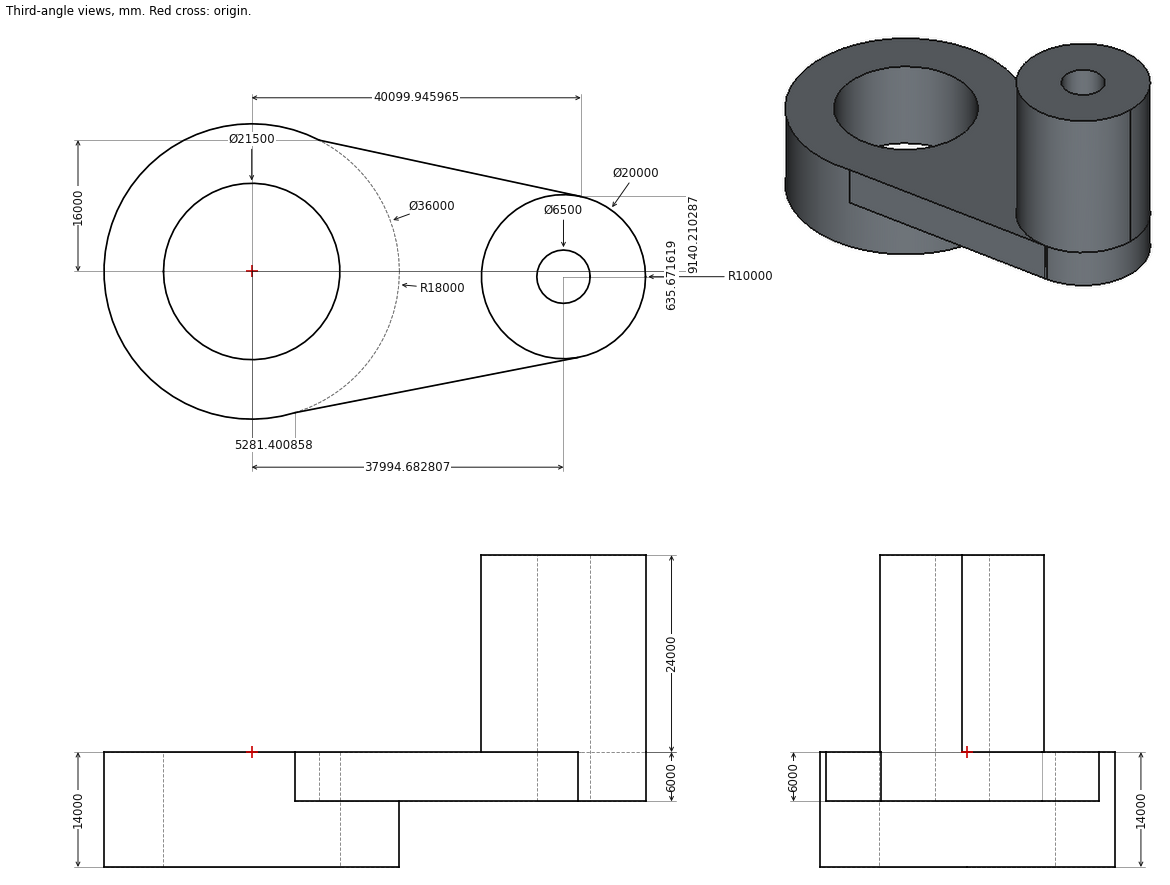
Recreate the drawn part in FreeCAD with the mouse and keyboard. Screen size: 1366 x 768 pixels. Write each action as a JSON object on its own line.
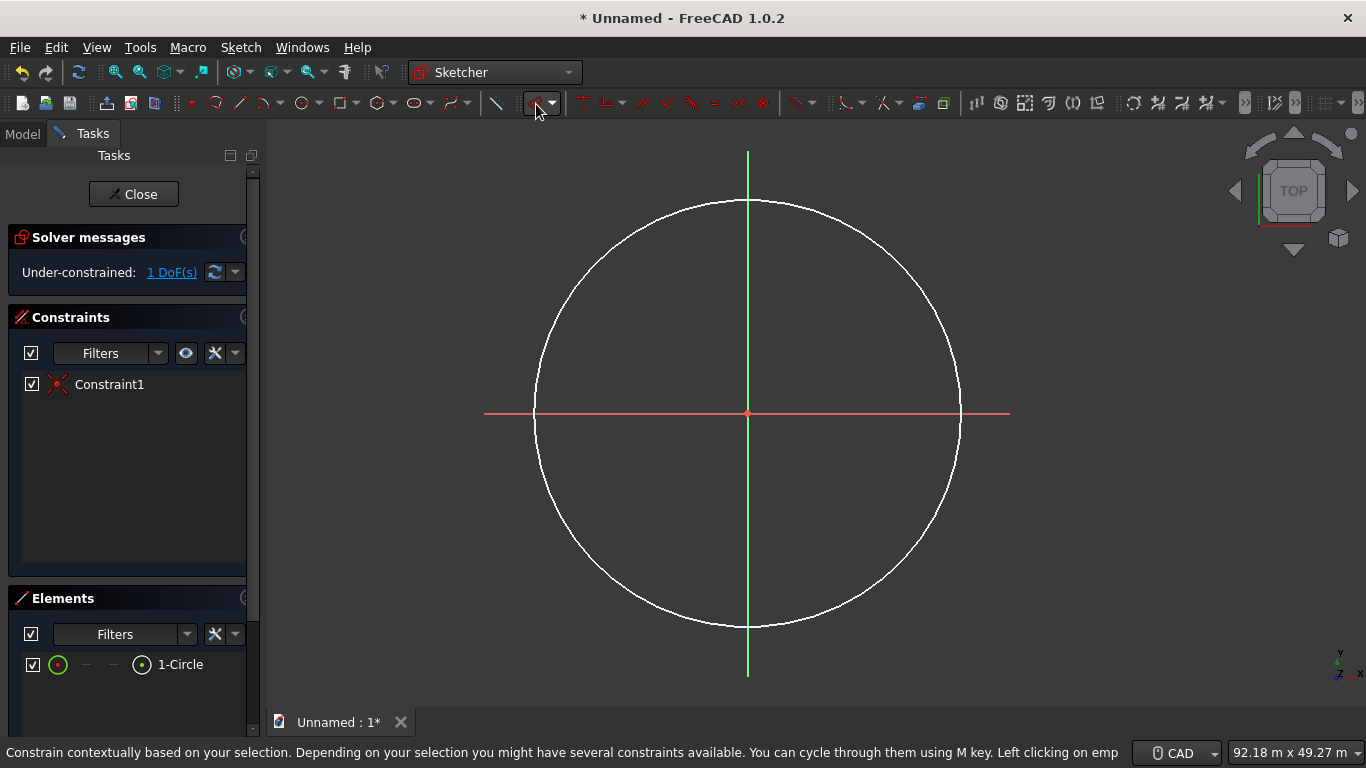
{"action": "left_click", "coordinate": [898, 262]}
{"action": "left_click", "coordinate": [921, 239]}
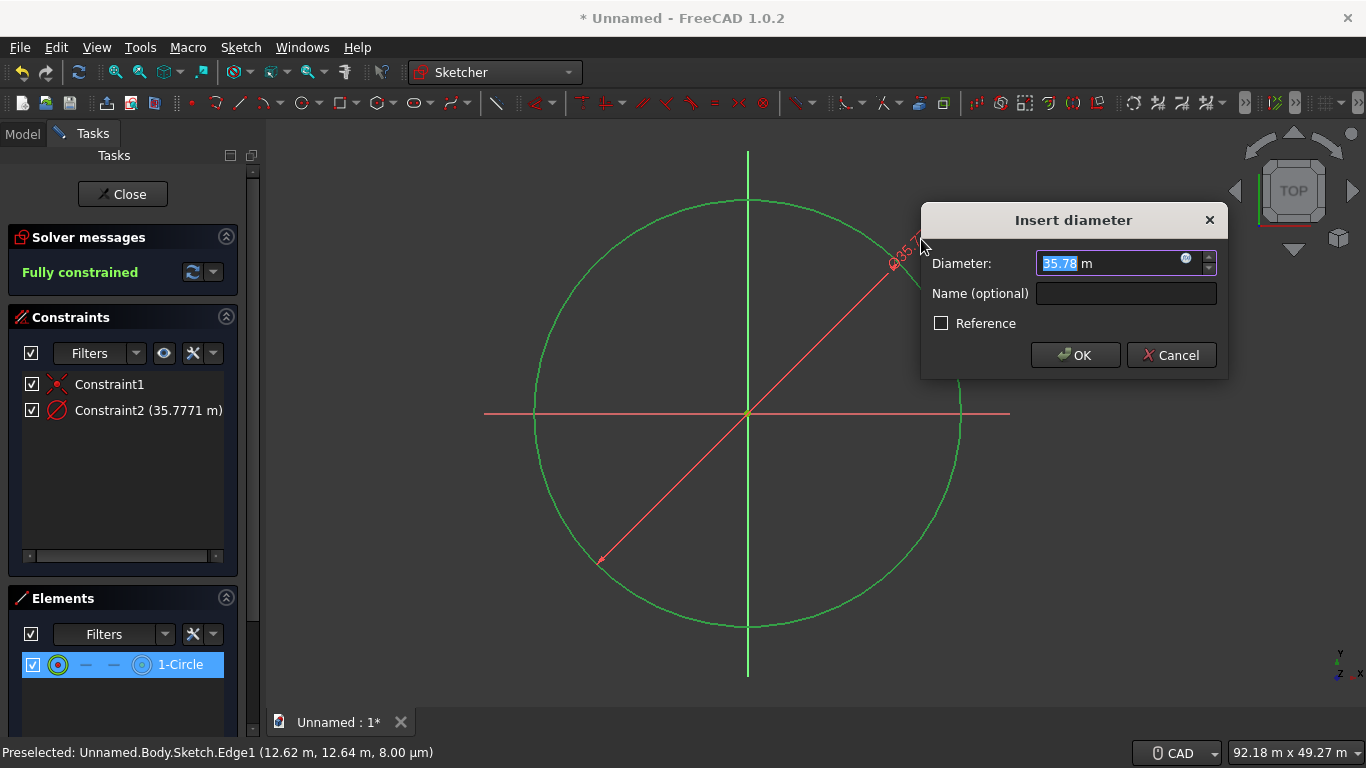
{"action": "key", "text": "ctrl+a"}
{"action": "type", "text": "36000 mm"}
{"action": "key", "text": "Return"}
{"action": "key", "text": "Escape"}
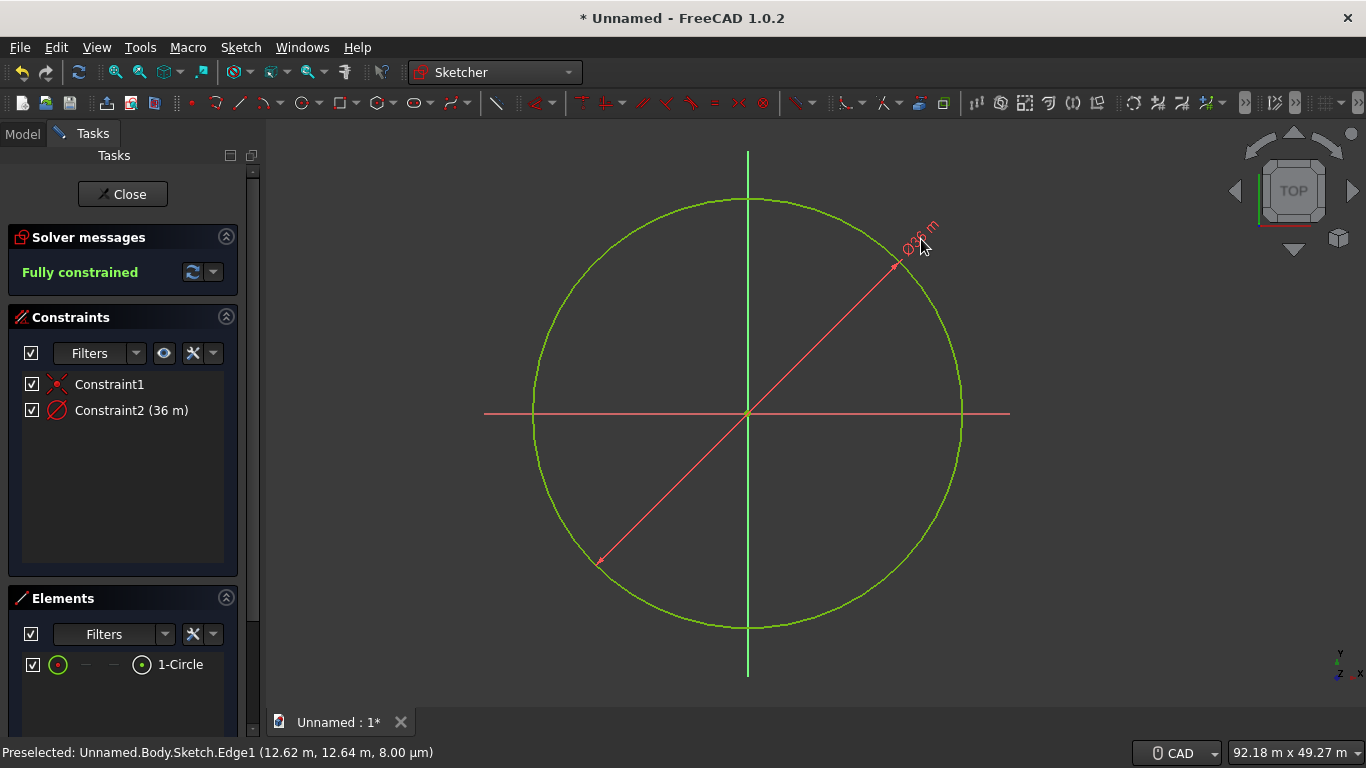
{"action": "left_click", "coordinate": [123, 194]}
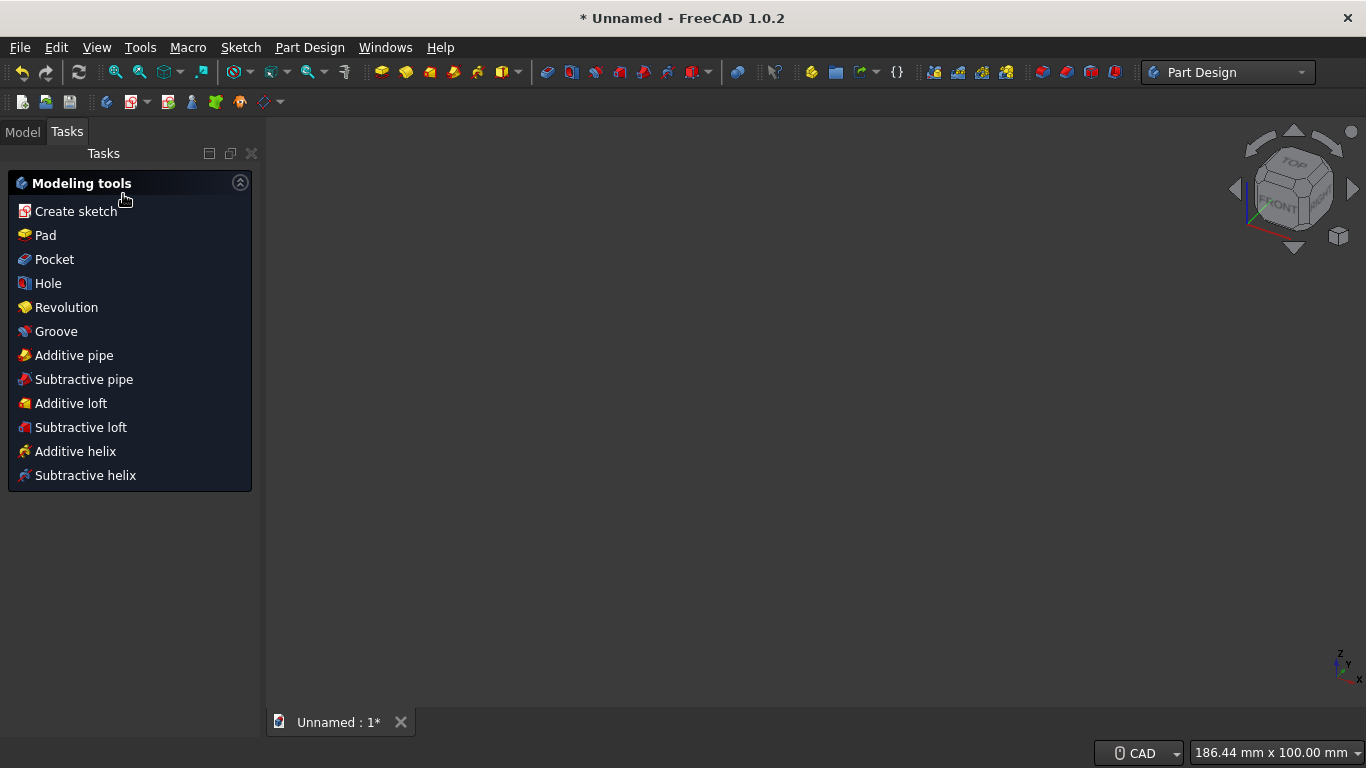
{"action": "left_click", "coordinate": [382, 72]}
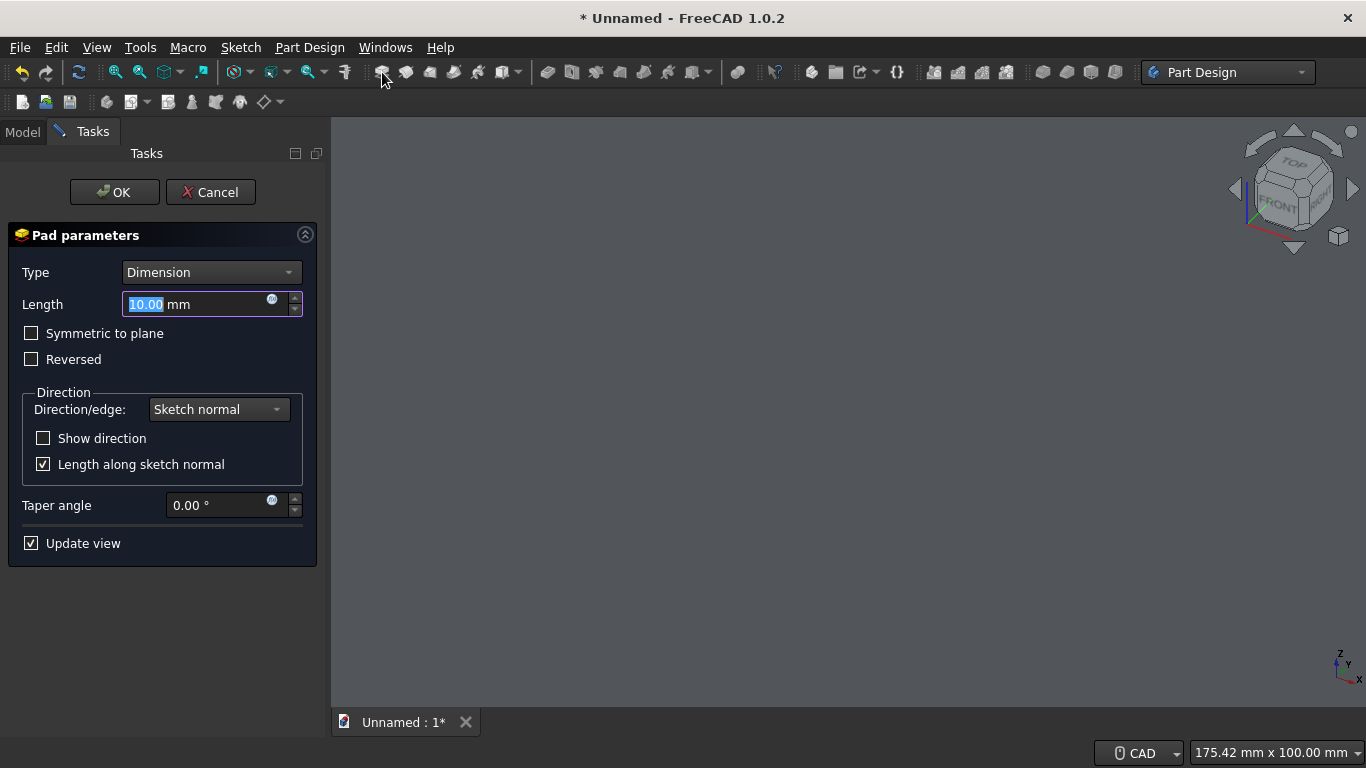
{"action": "type", "text": "14000"}
{"action": "key", "text": "Tab"}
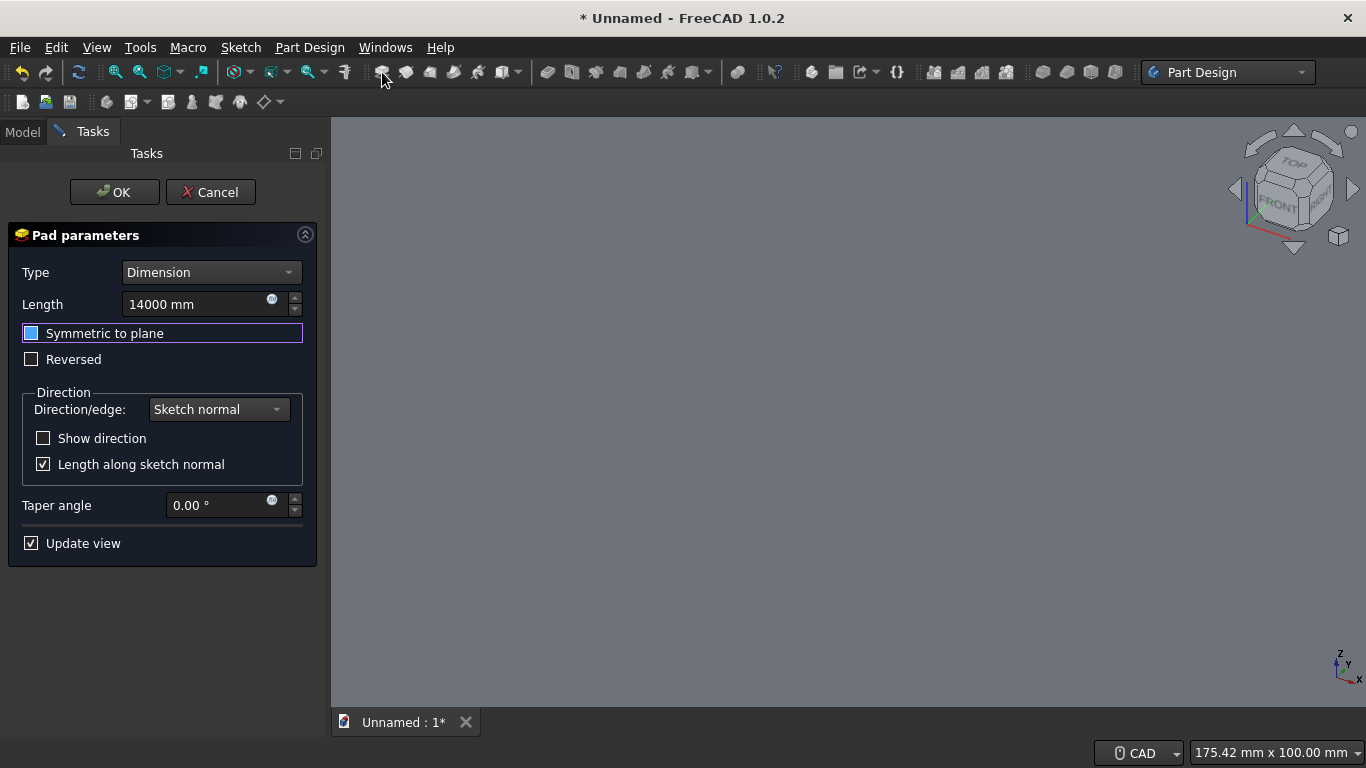
{"action": "left_click", "coordinate": [30, 359]}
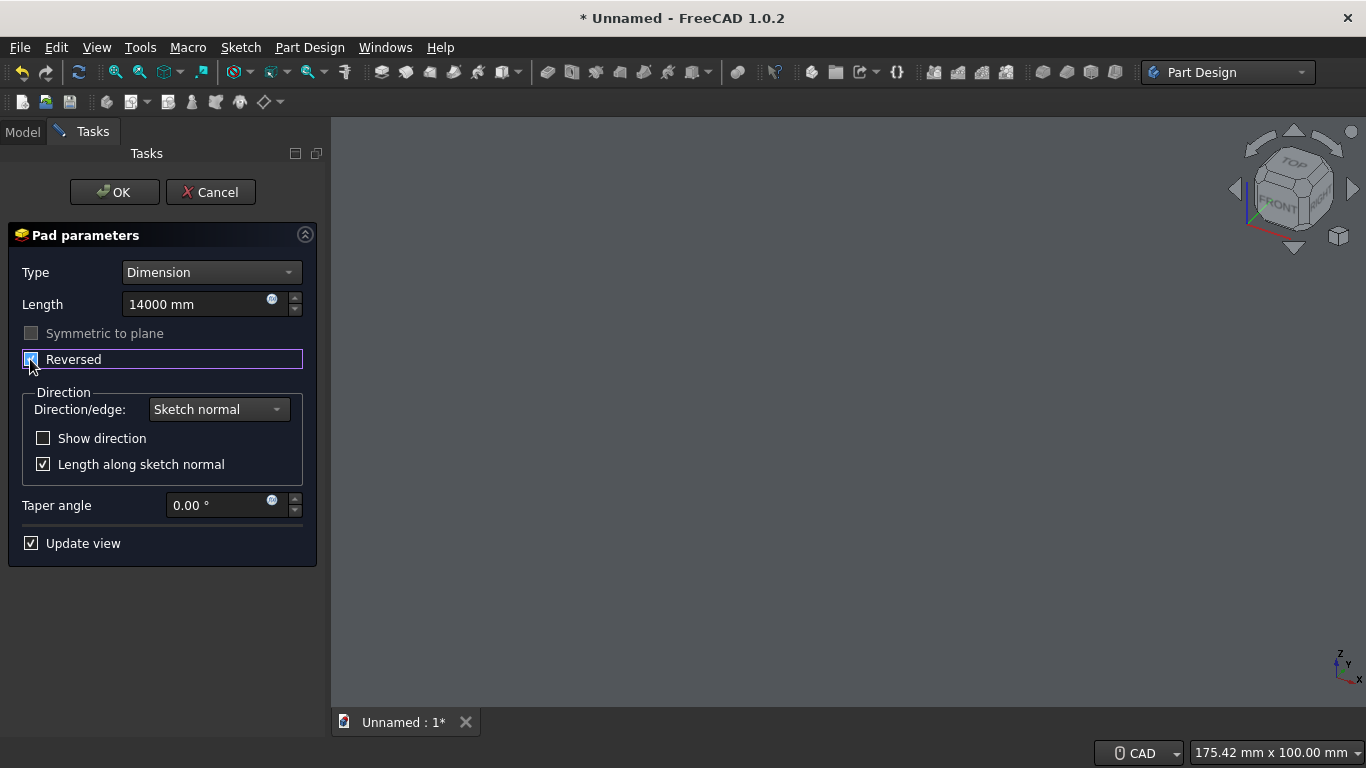
{"action": "left_click", "coordinate": [115, 192]}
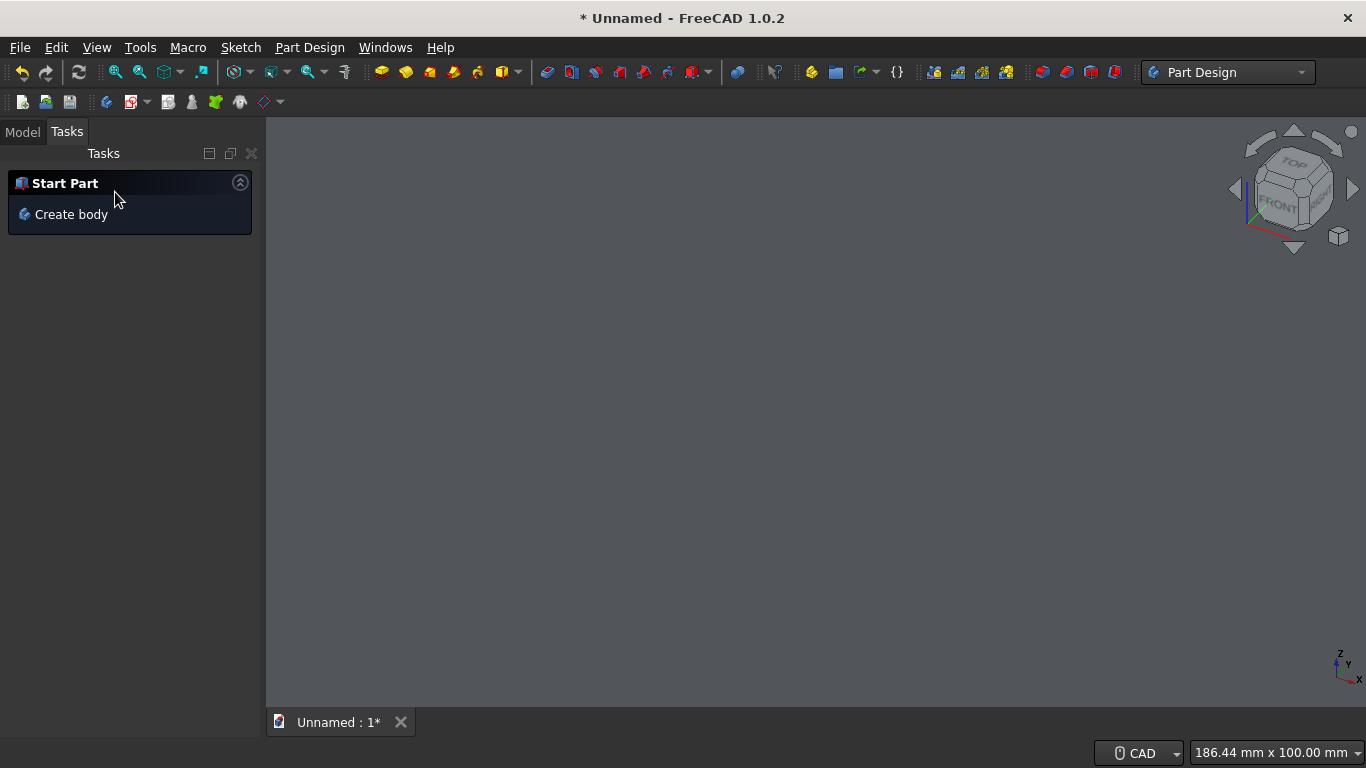
{"action": "left_click", "coordinate": [116, 72]}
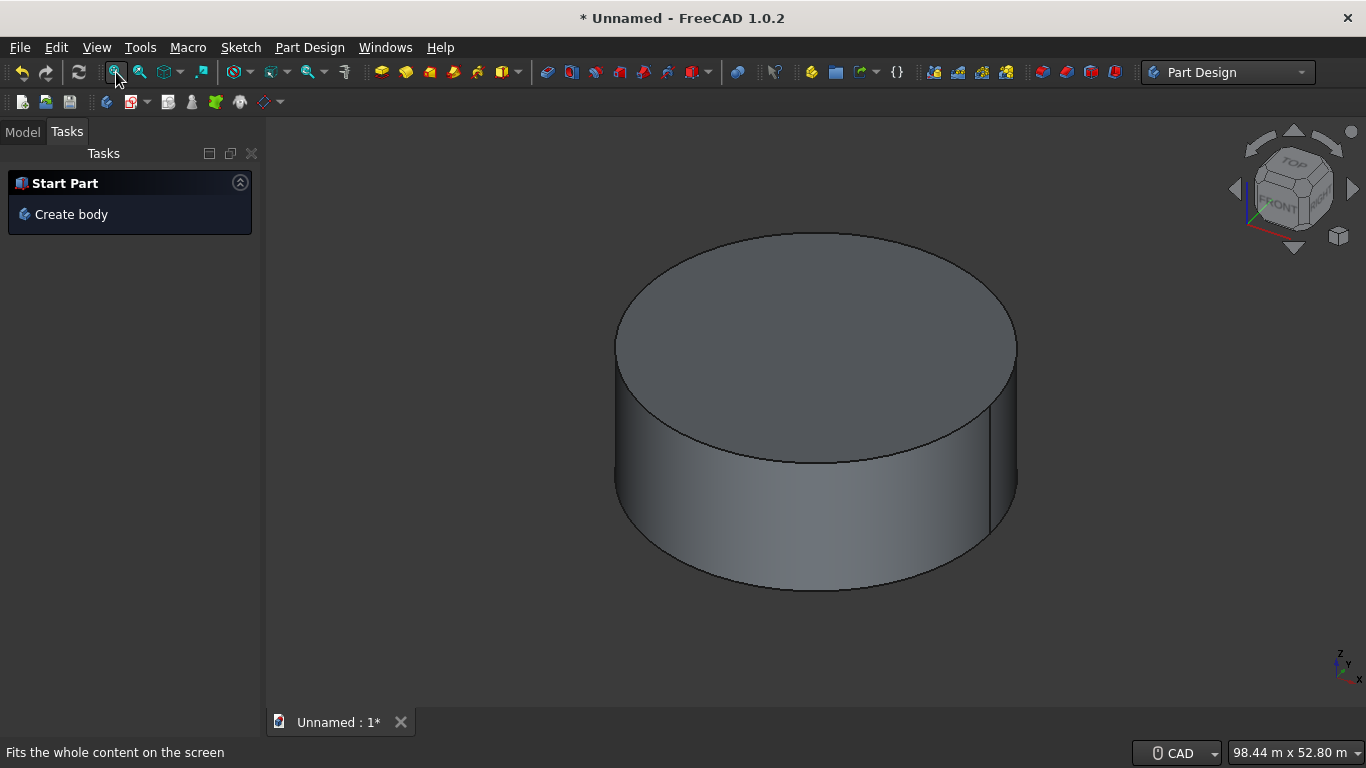
{"action": "key", "text": "5"}